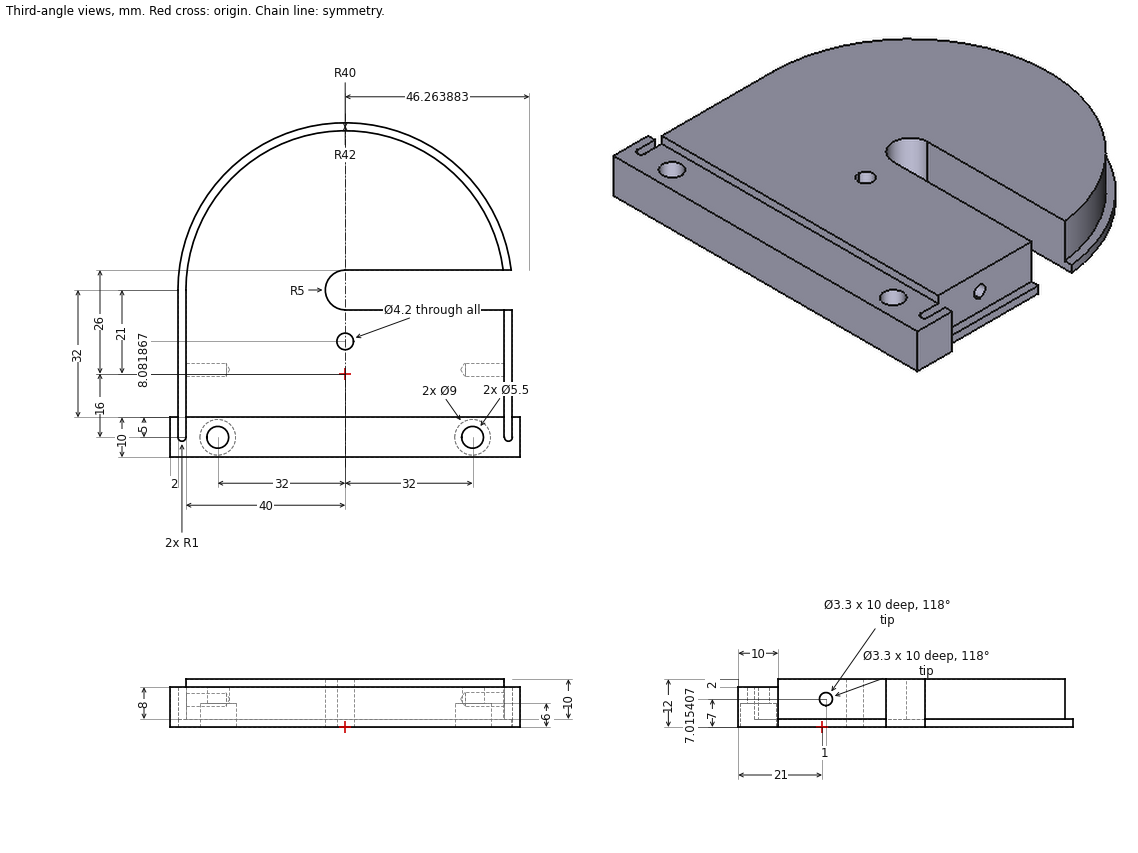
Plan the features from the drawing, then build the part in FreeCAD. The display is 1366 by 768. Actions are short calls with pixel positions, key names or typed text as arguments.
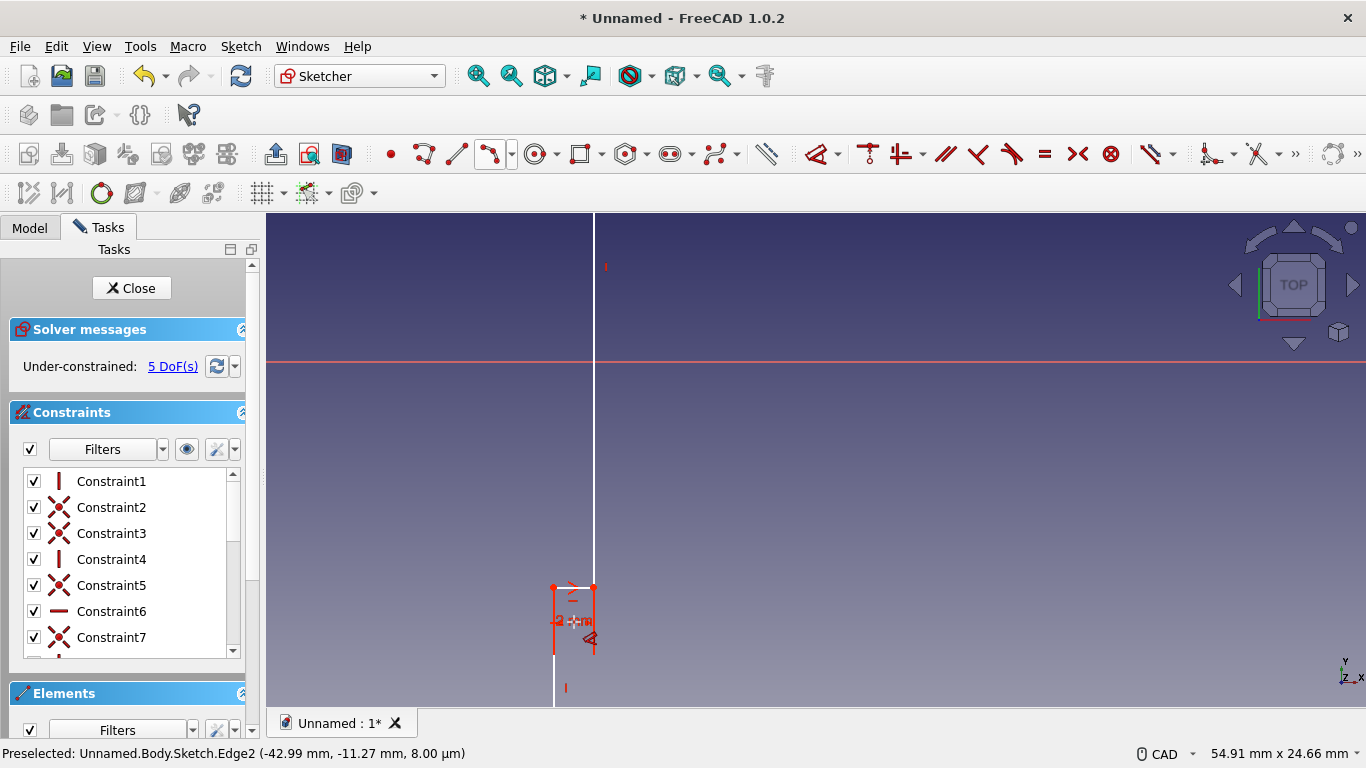
click(594, 395)
click(560, 414)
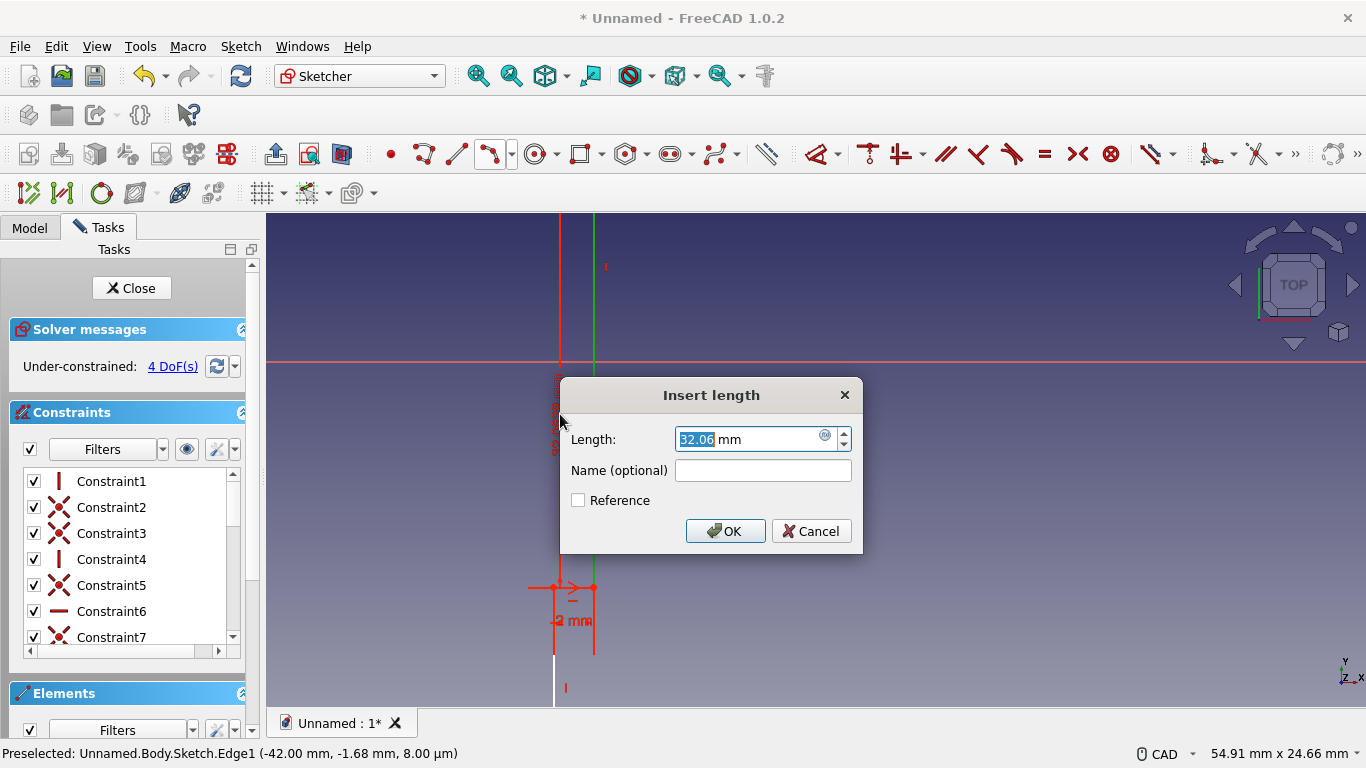
text(32)
key(Return)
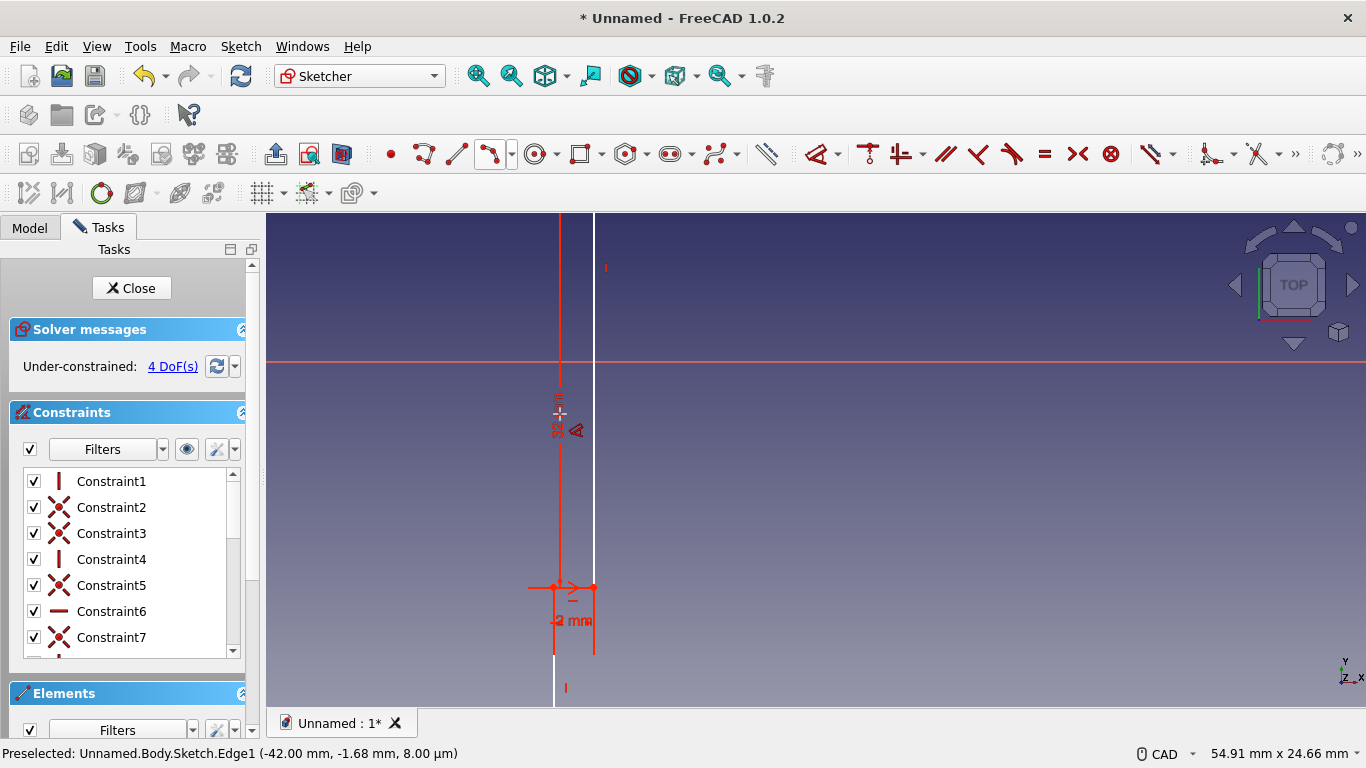
scroll(574, 591, down, 8)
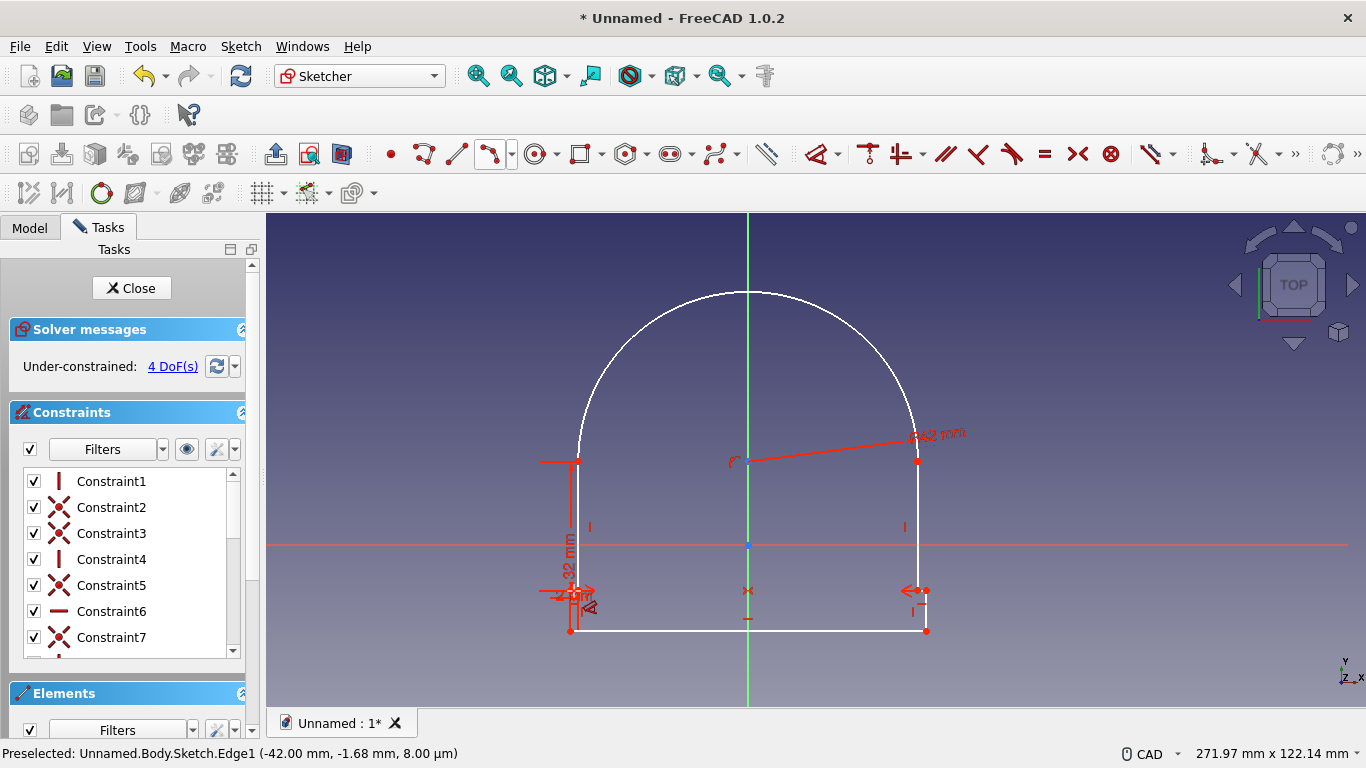
click(570, 603)
click(536, 620)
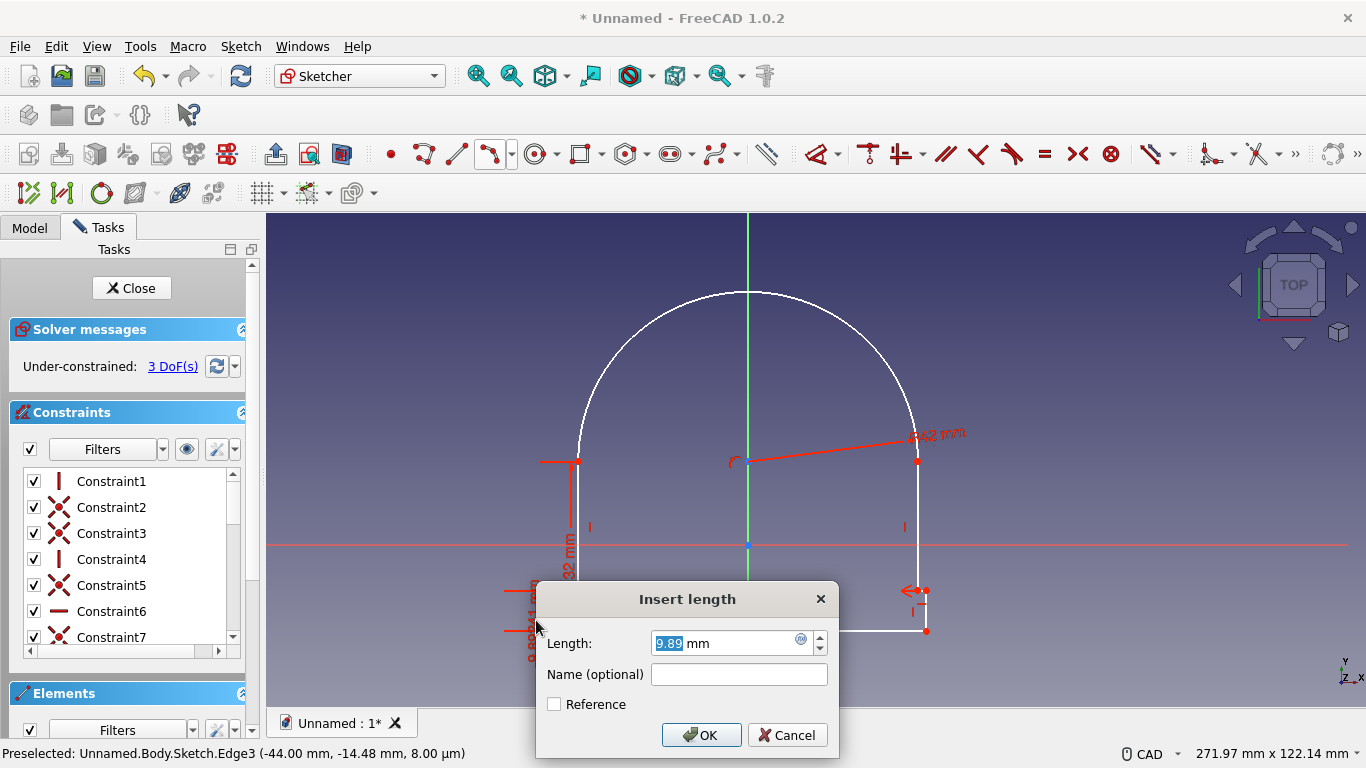
text(10)
key(Return)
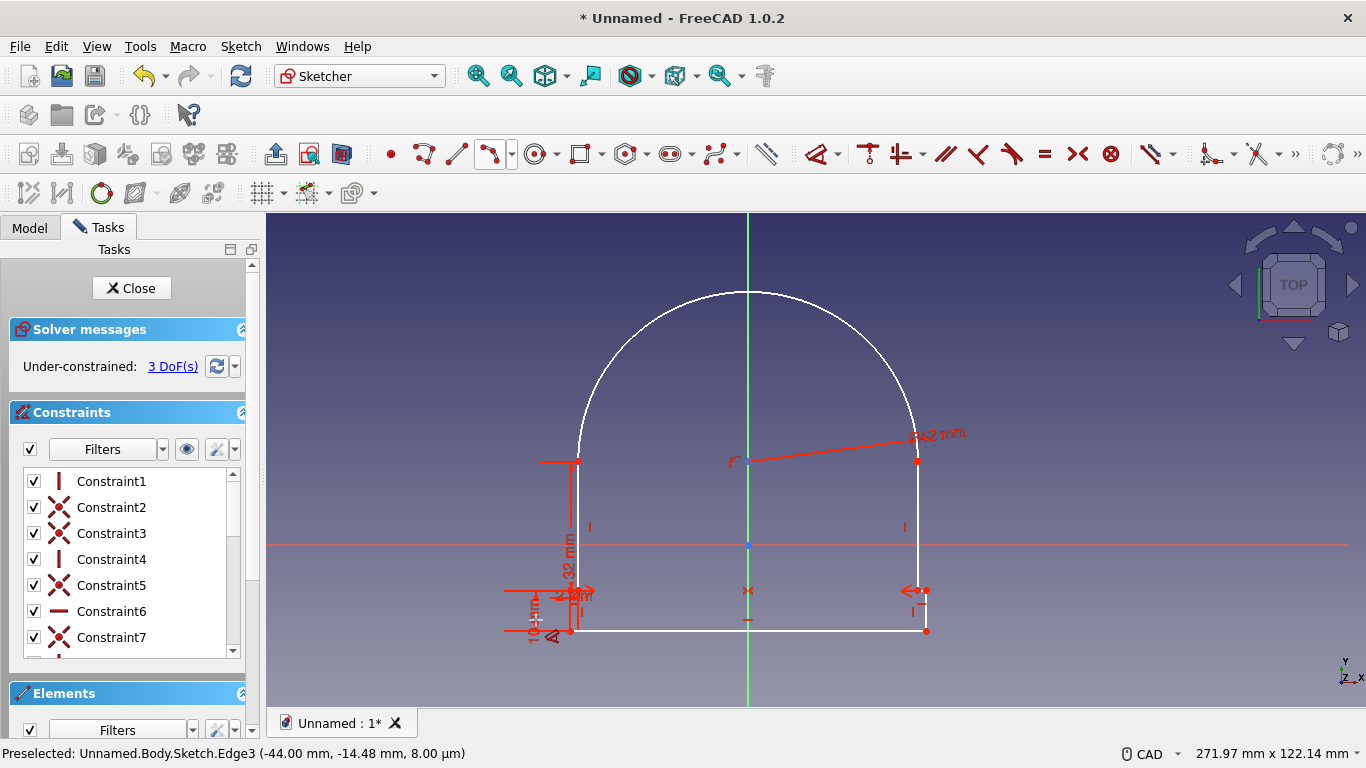
click(918, 500)
click(952, 526)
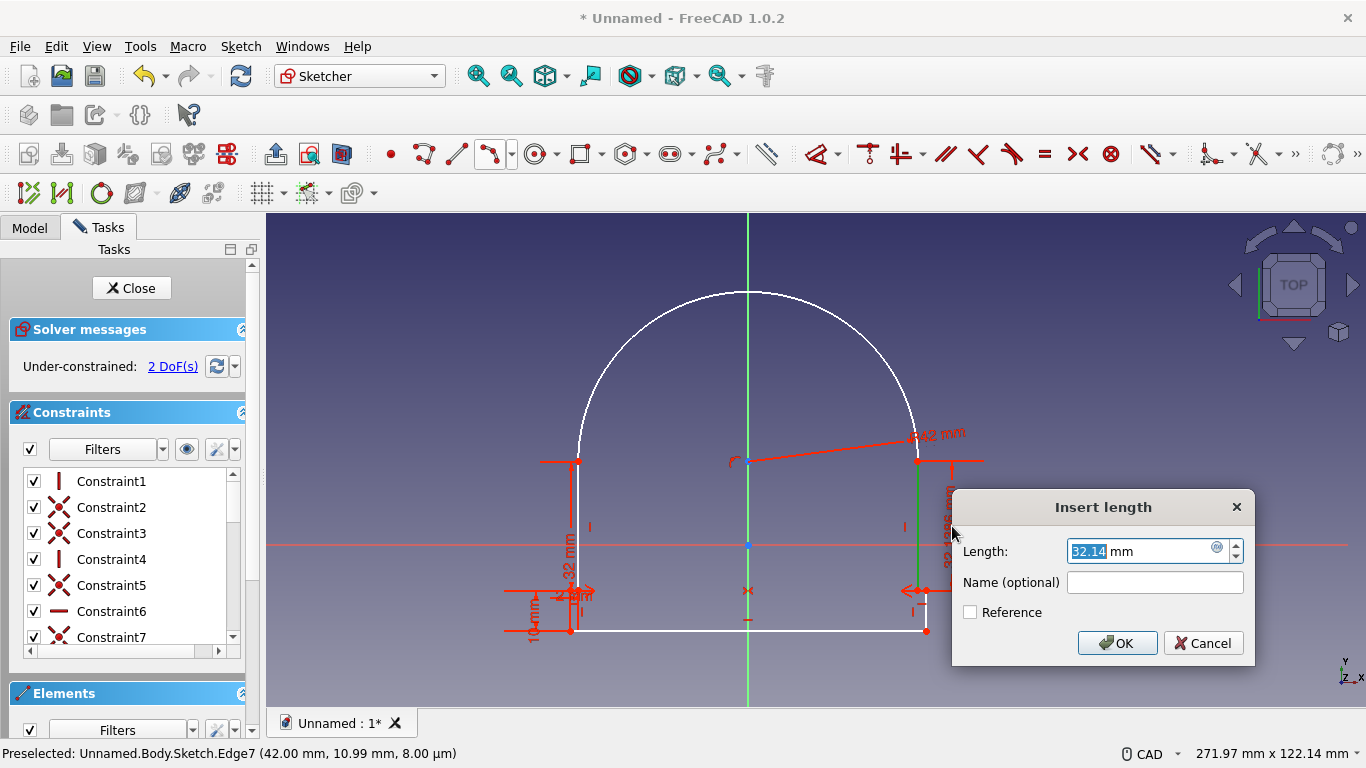
text(32)
key(Return)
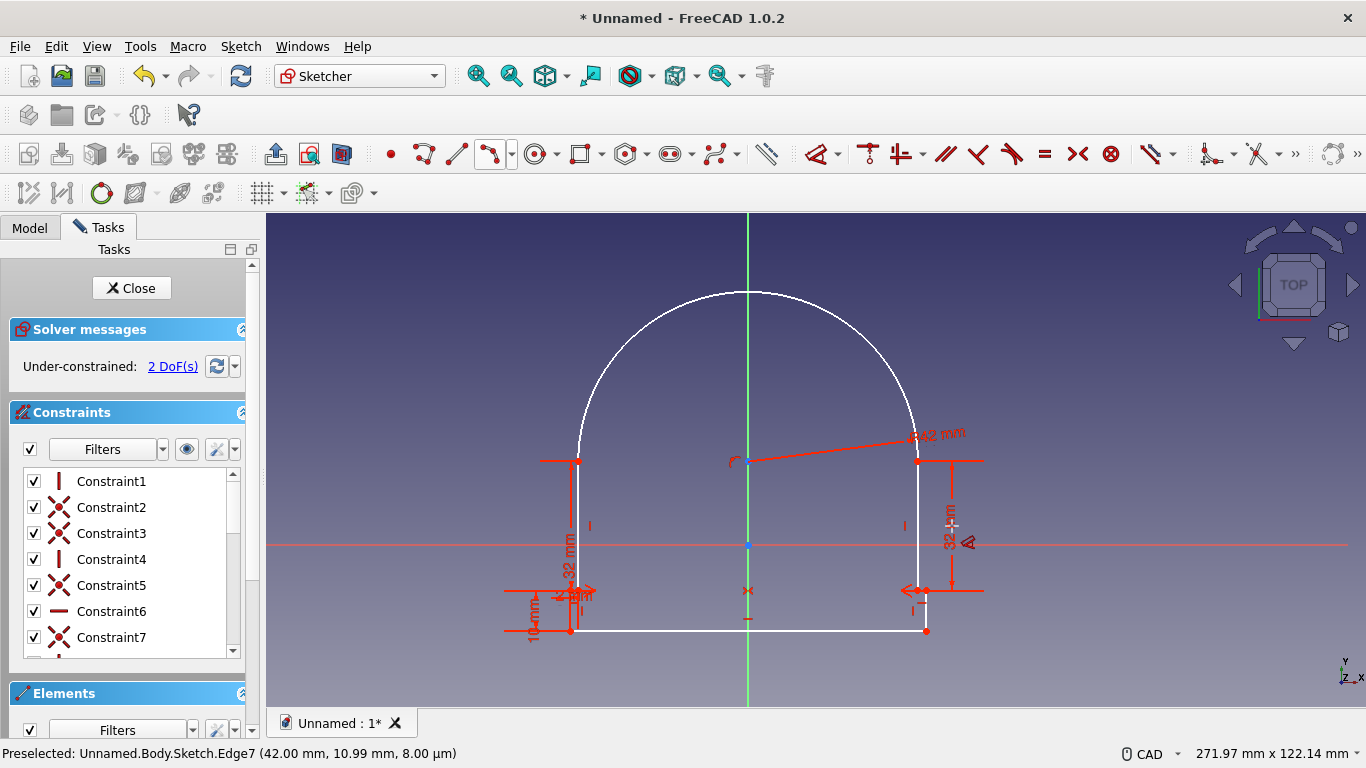
click(578, 461)
click(544, 503)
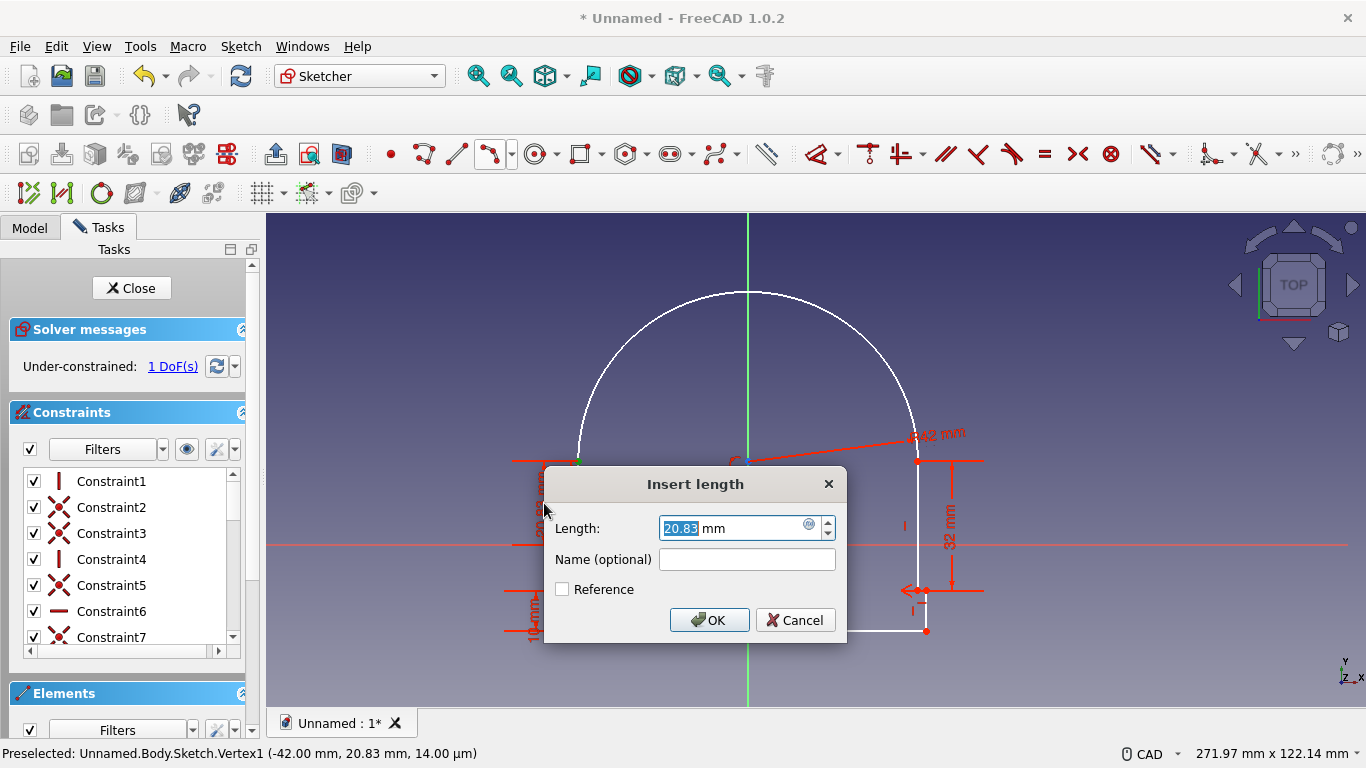
text(21)
key(Return)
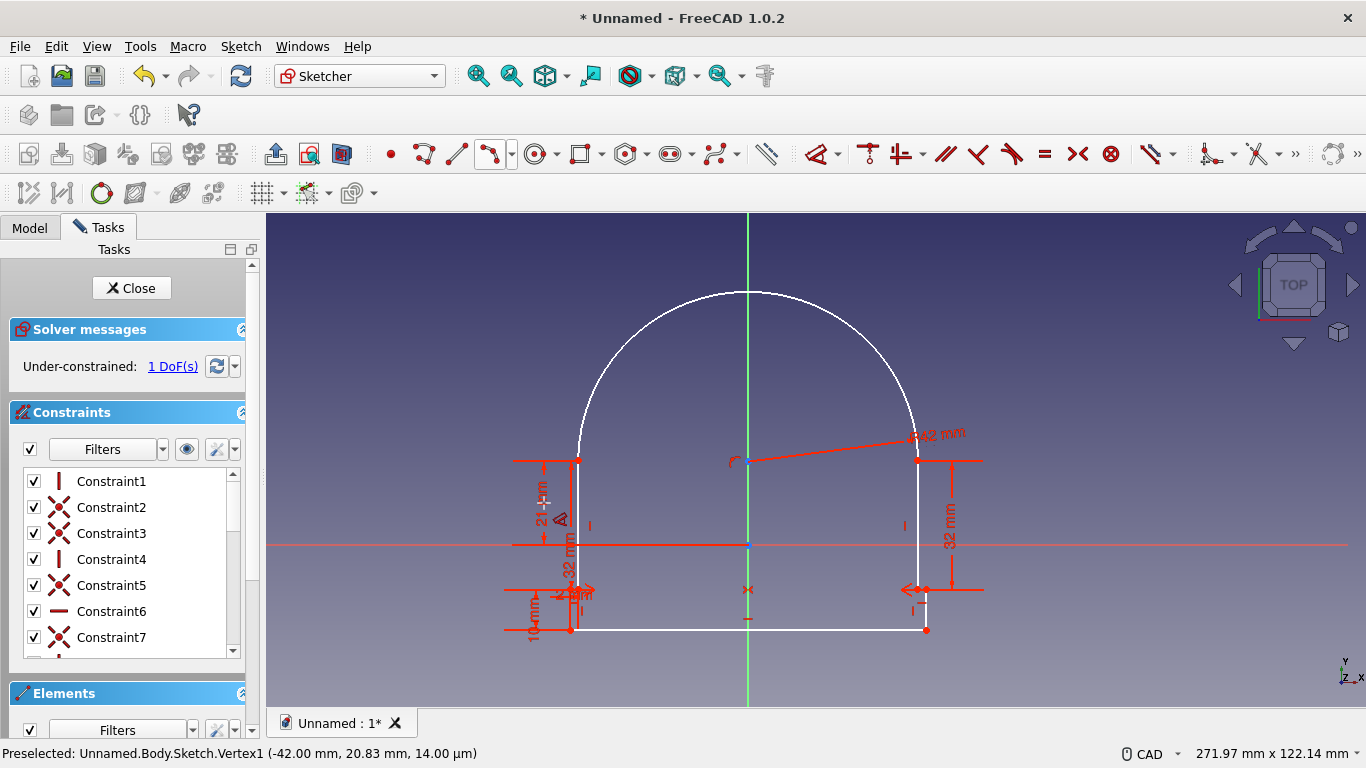
click(748, 462)
click(782, 504)